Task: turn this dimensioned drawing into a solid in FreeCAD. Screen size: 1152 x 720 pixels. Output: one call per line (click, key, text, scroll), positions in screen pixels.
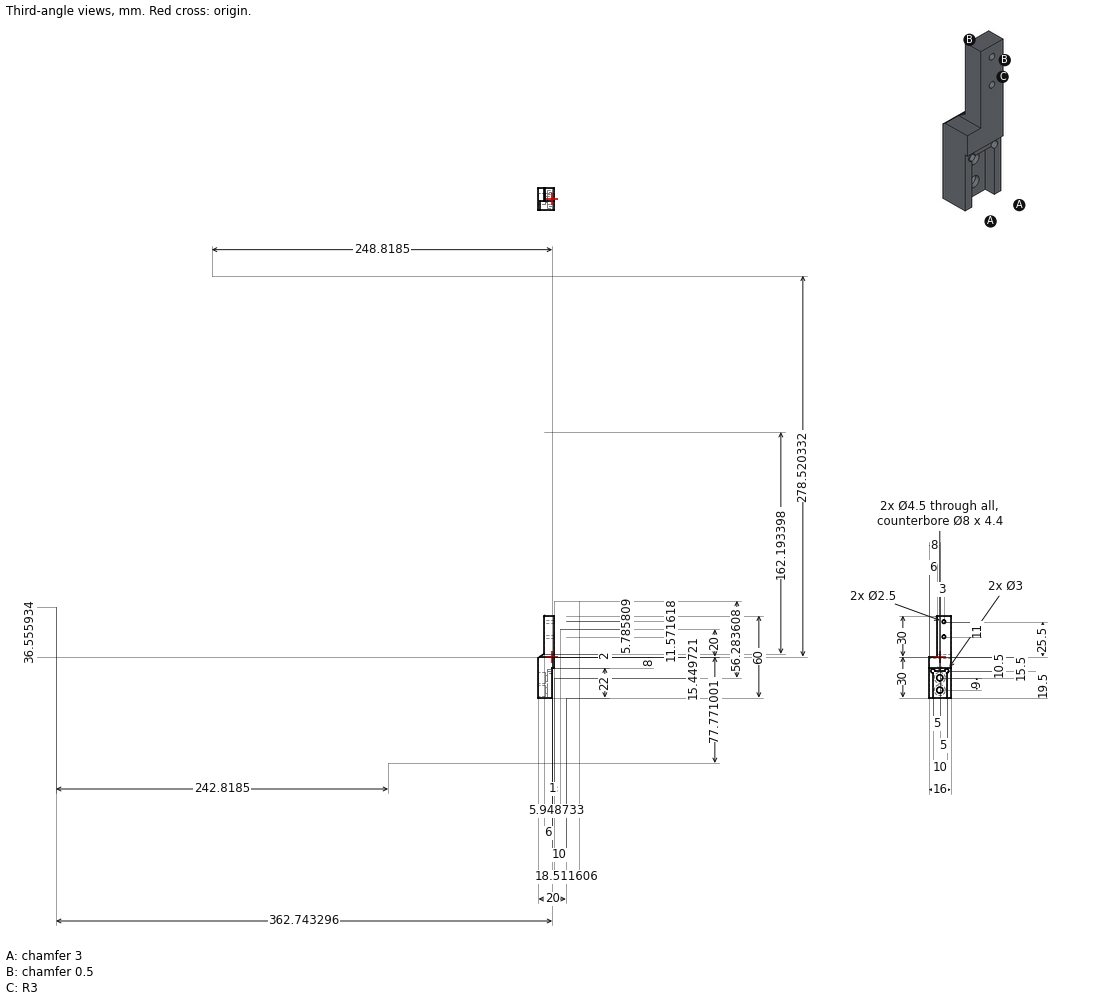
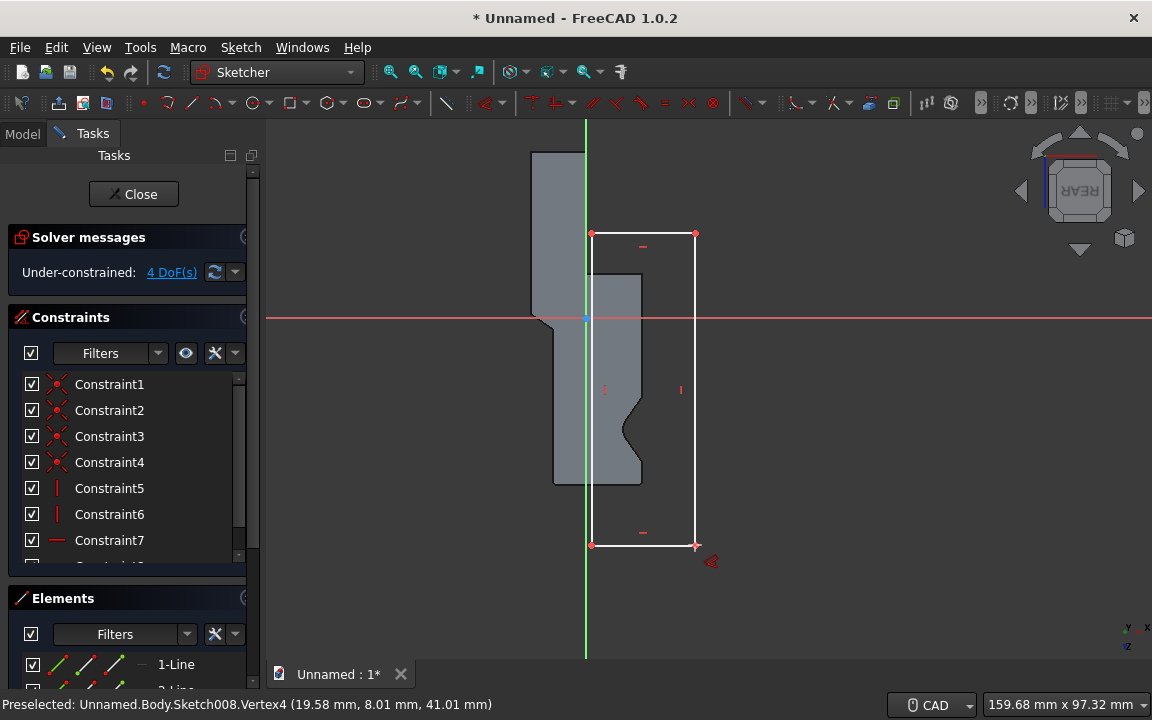
scroll(592, 233, up, 10)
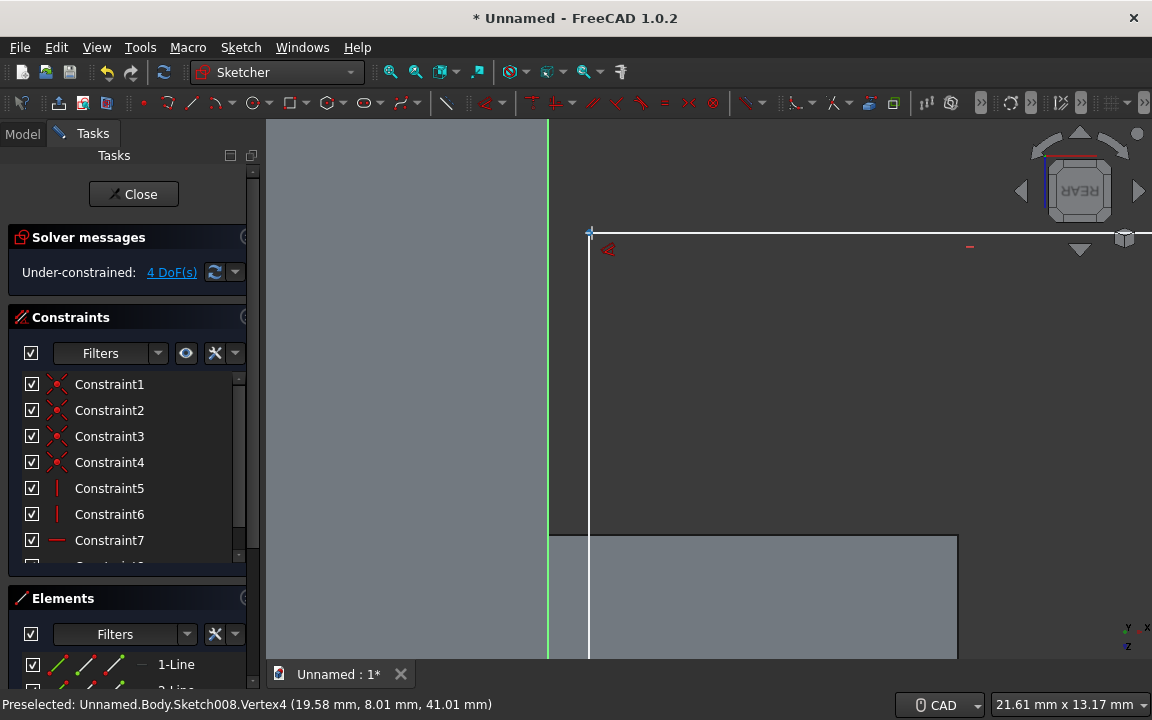
click(589, 233)
click(569, 199)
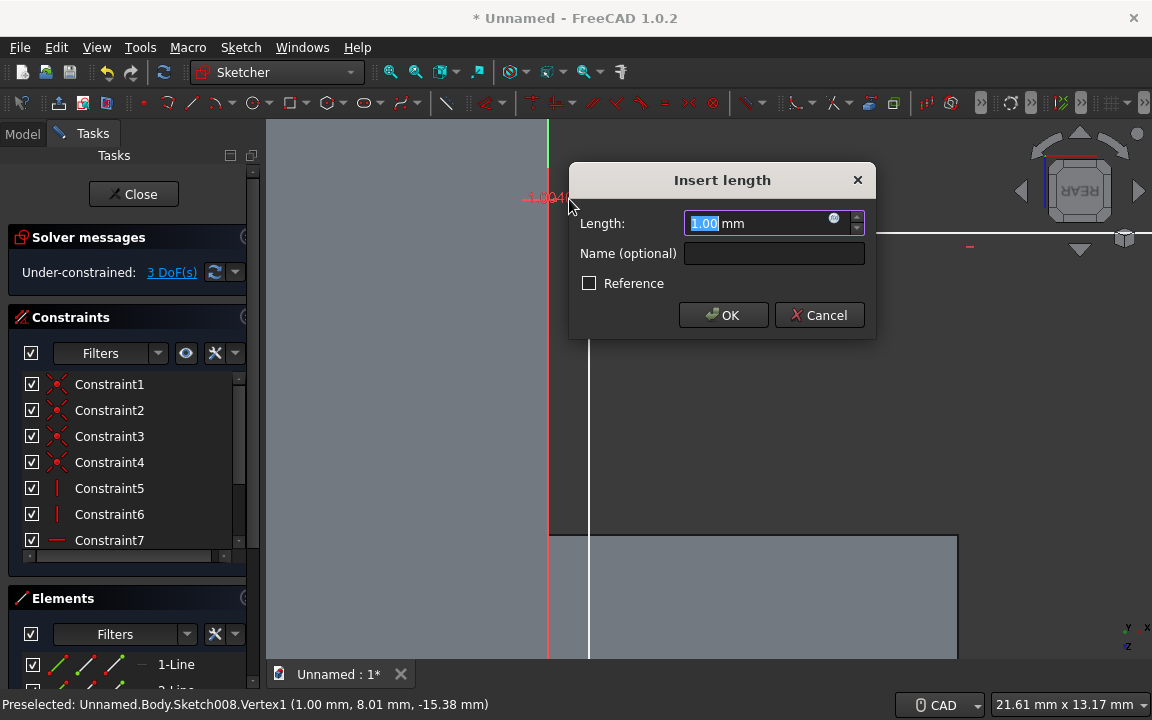
text(1)
key(Return)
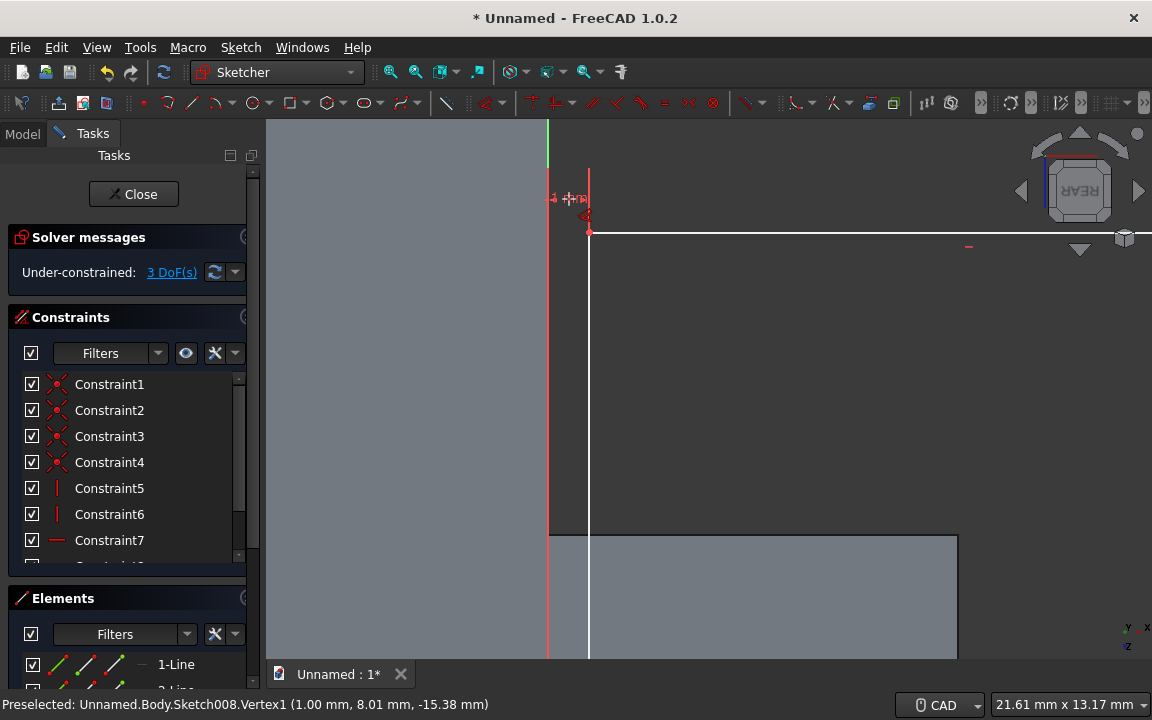
scroll(592, 233, down, 10)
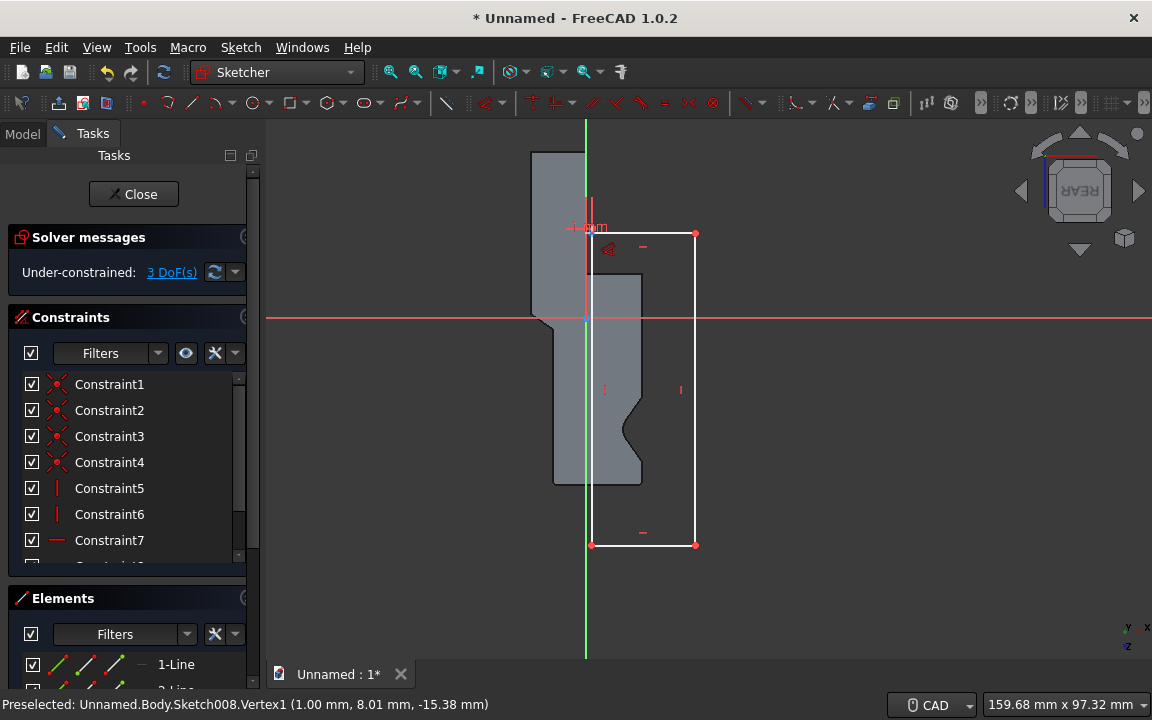
scroll(592, 327, up, 5)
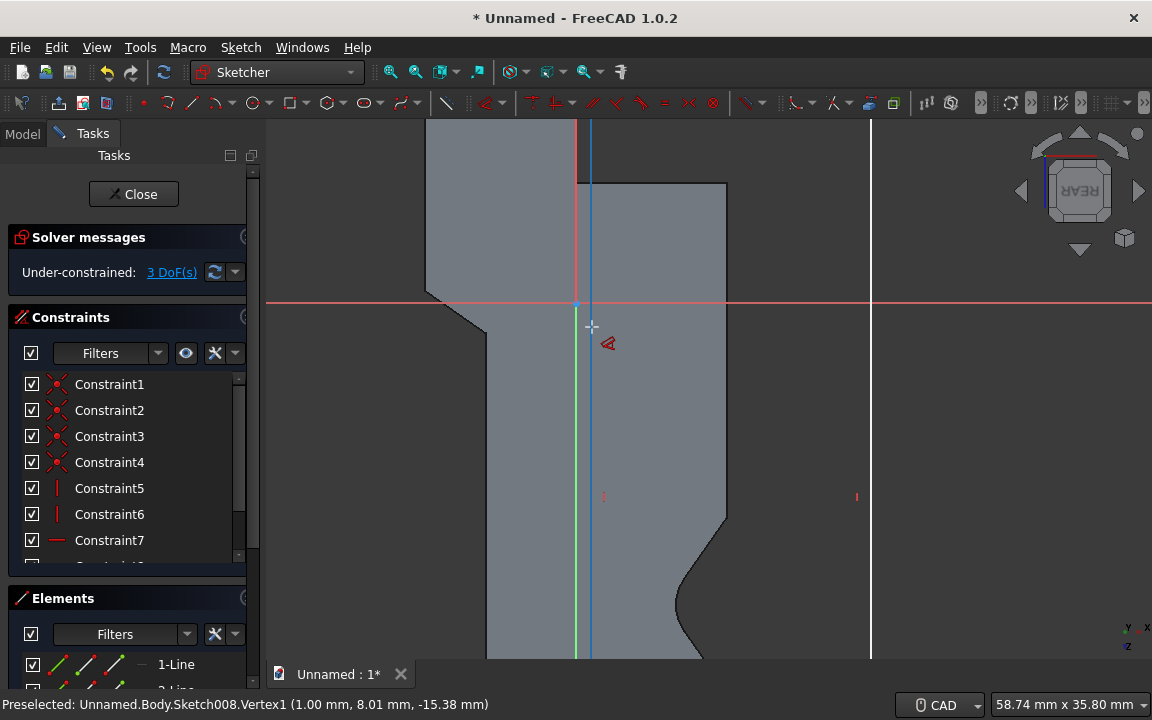
click(591, 326)
click(557, 389)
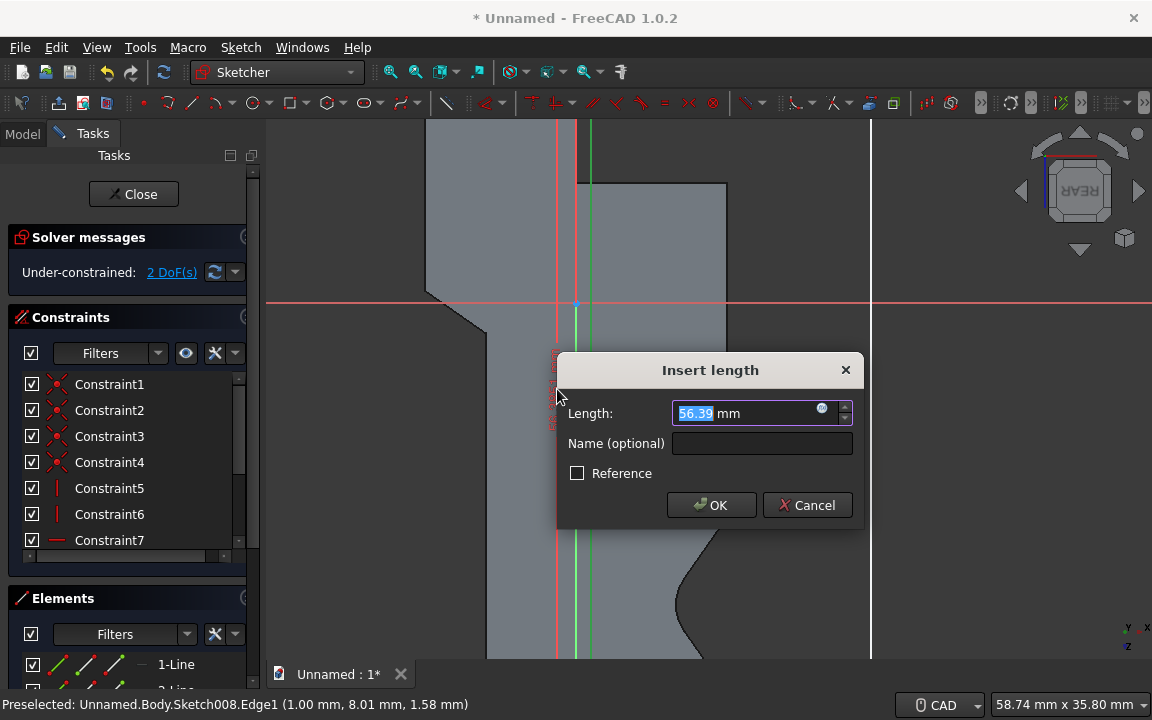
text(56.283608)
key(Return)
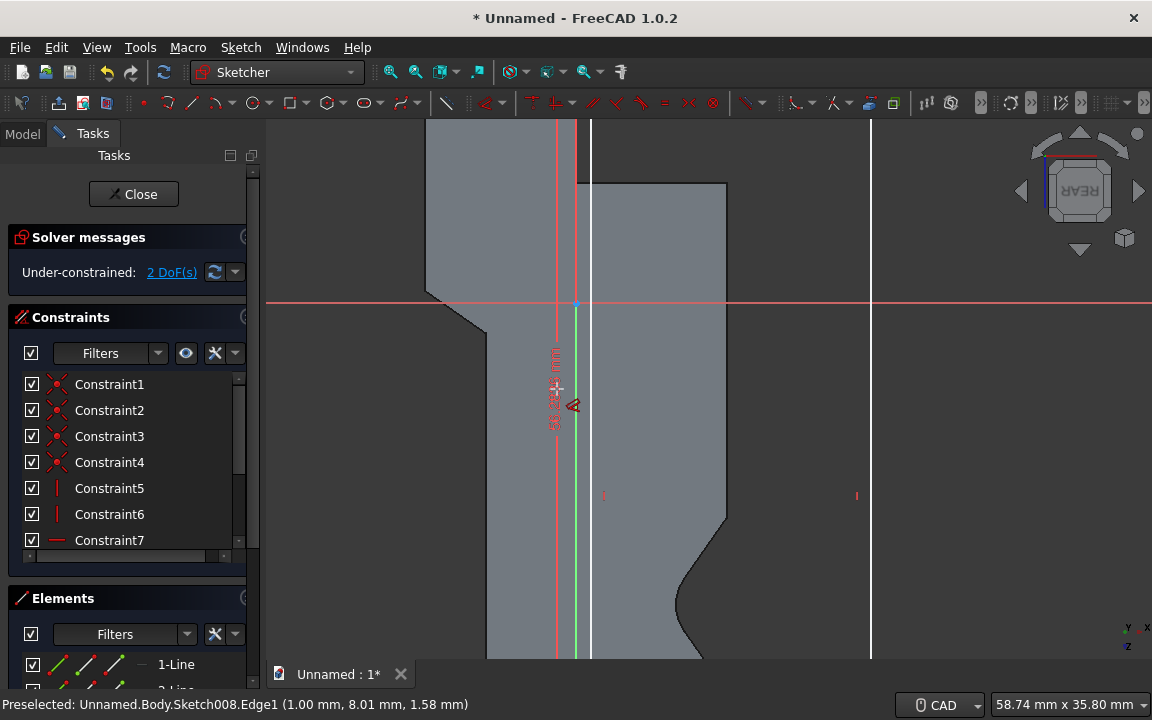
scroll(592, 328, down, 5)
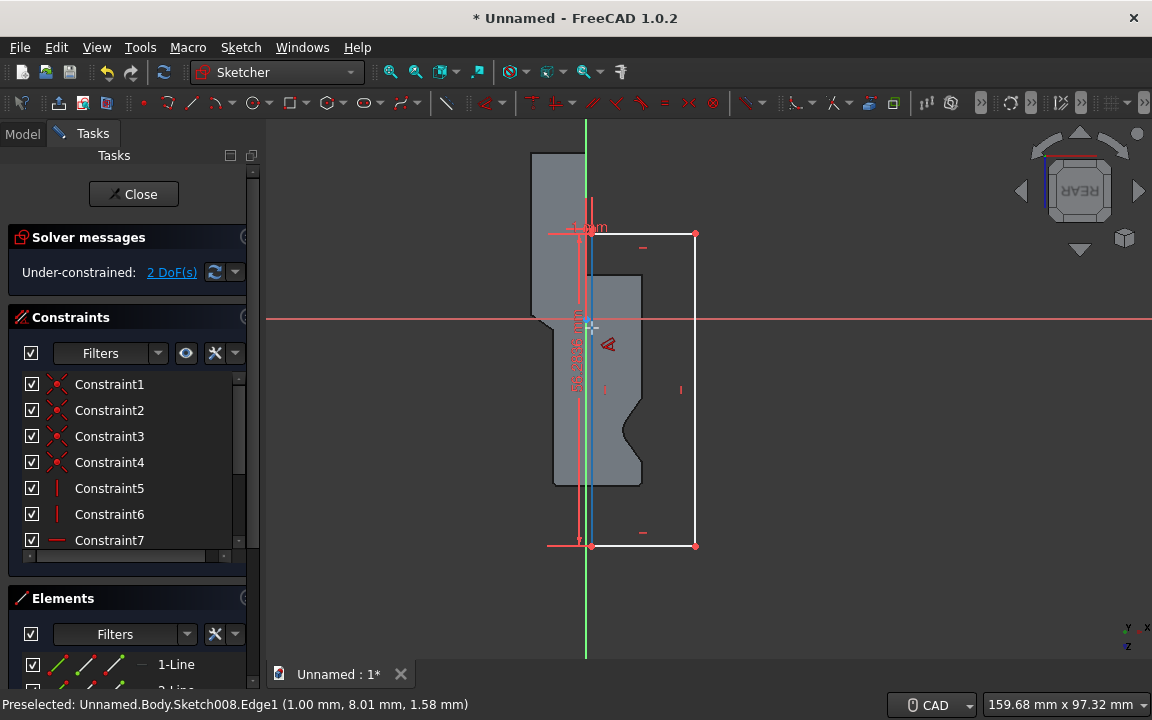
click(623, 546)
click(643, 580)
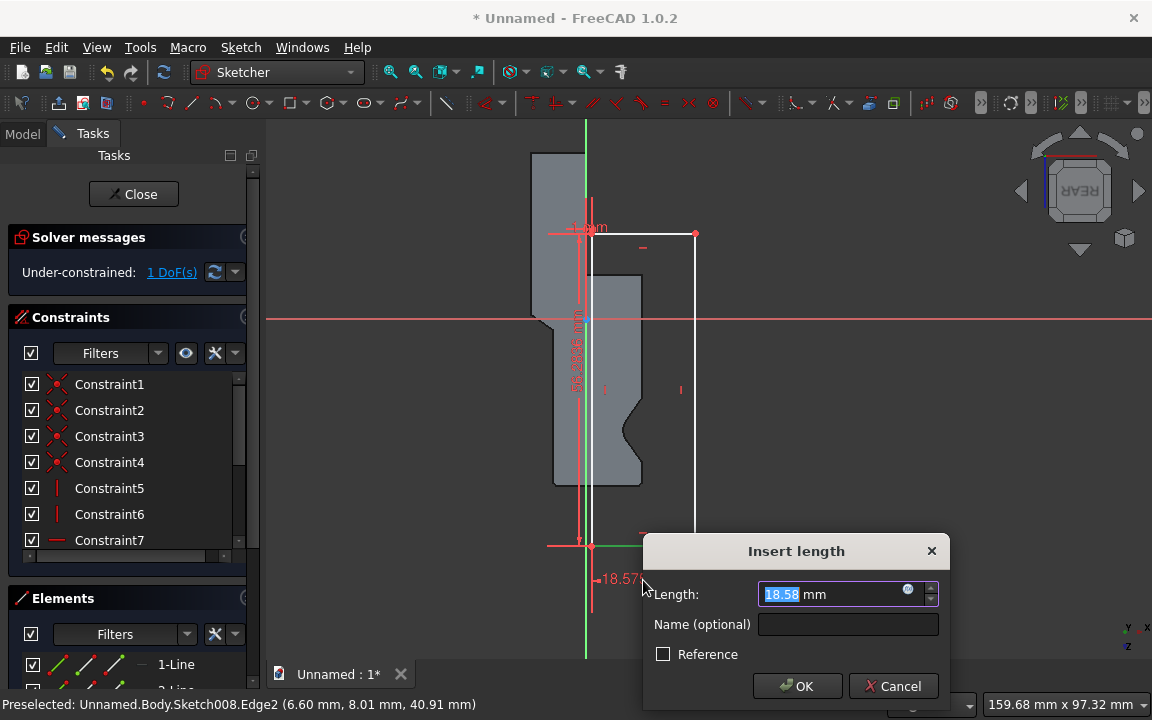
text(18.511606)
key(Return)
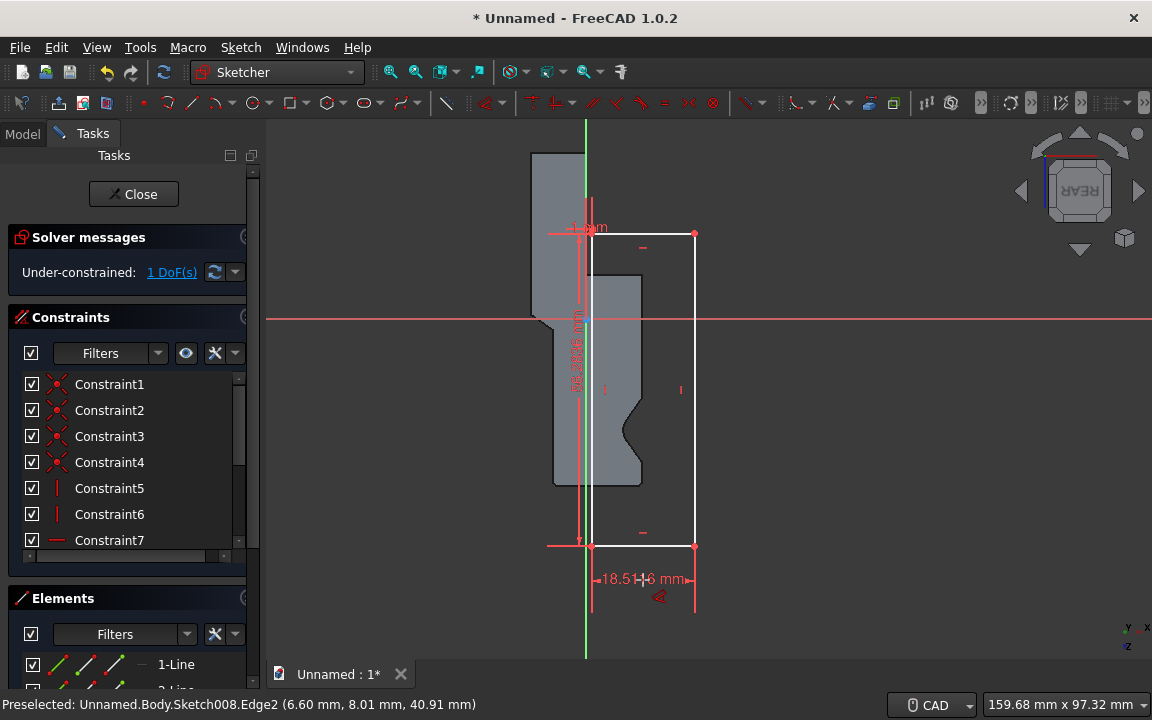
click(592, 234)
click(552, 276)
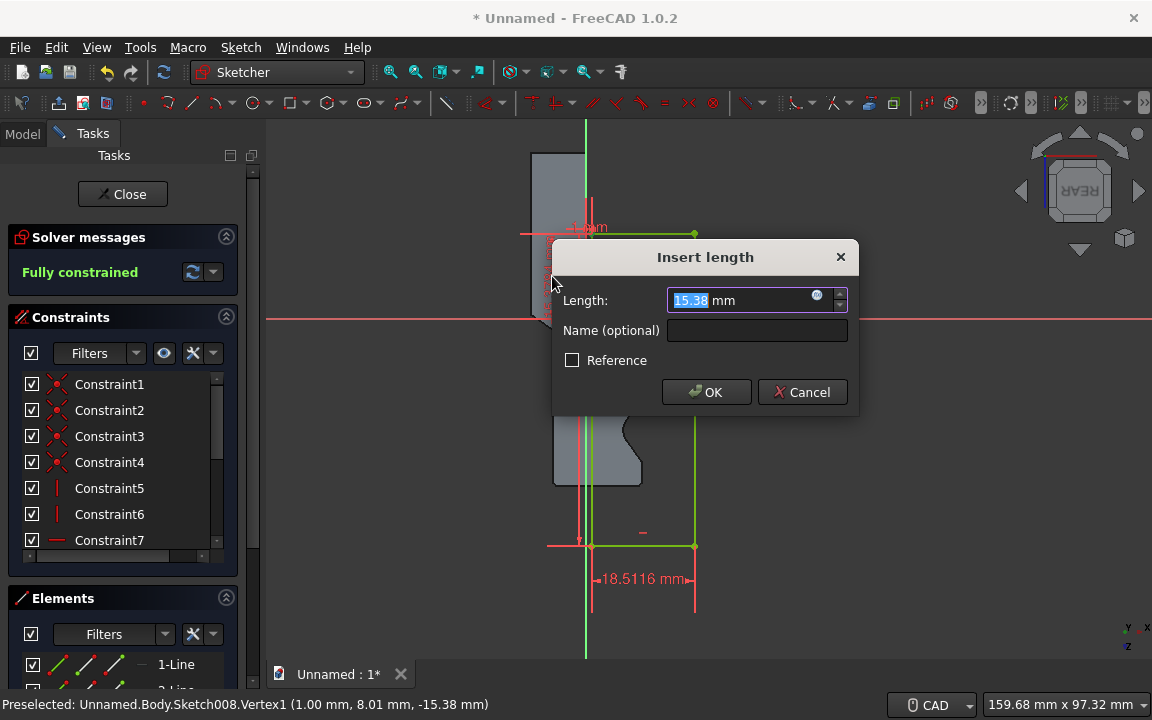
text(15.449721)
key(Return)
key(Escape)